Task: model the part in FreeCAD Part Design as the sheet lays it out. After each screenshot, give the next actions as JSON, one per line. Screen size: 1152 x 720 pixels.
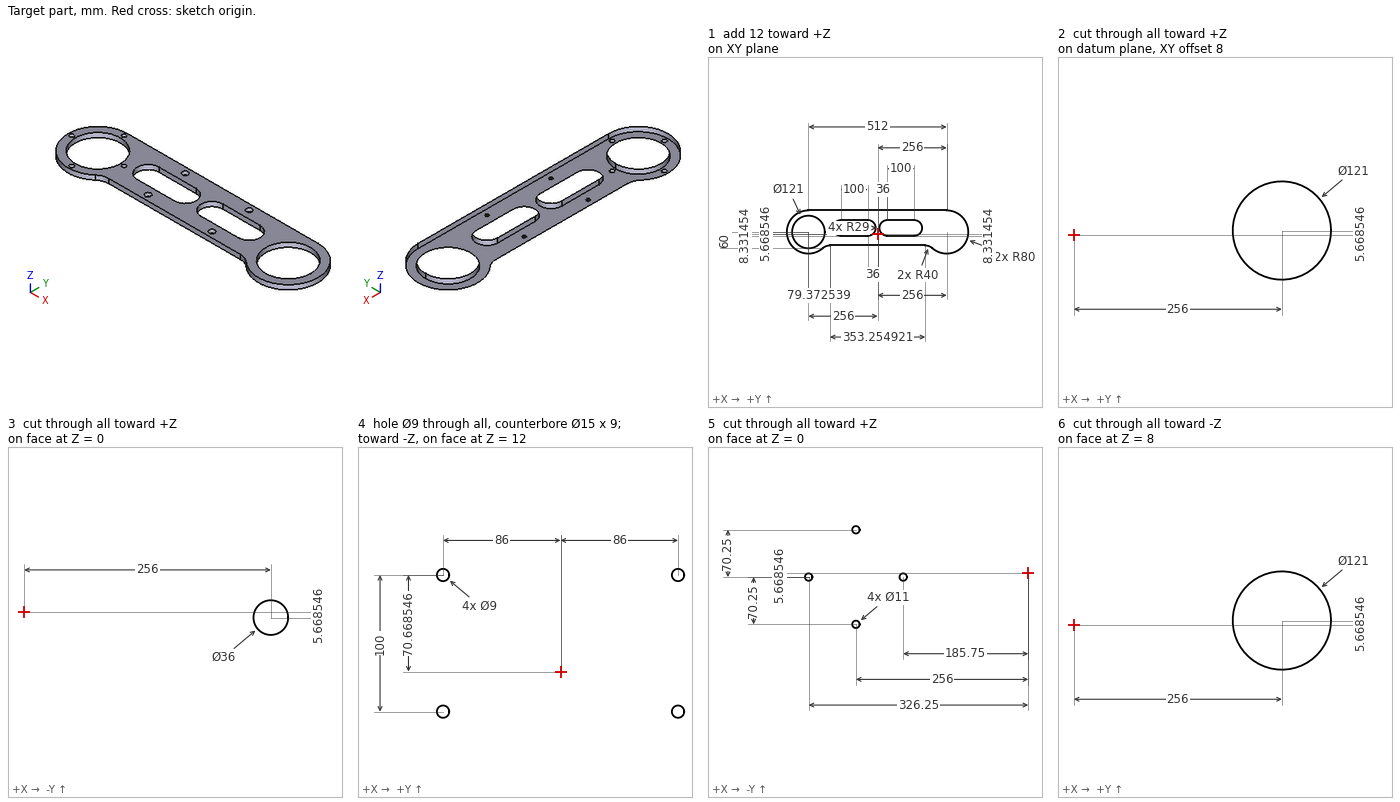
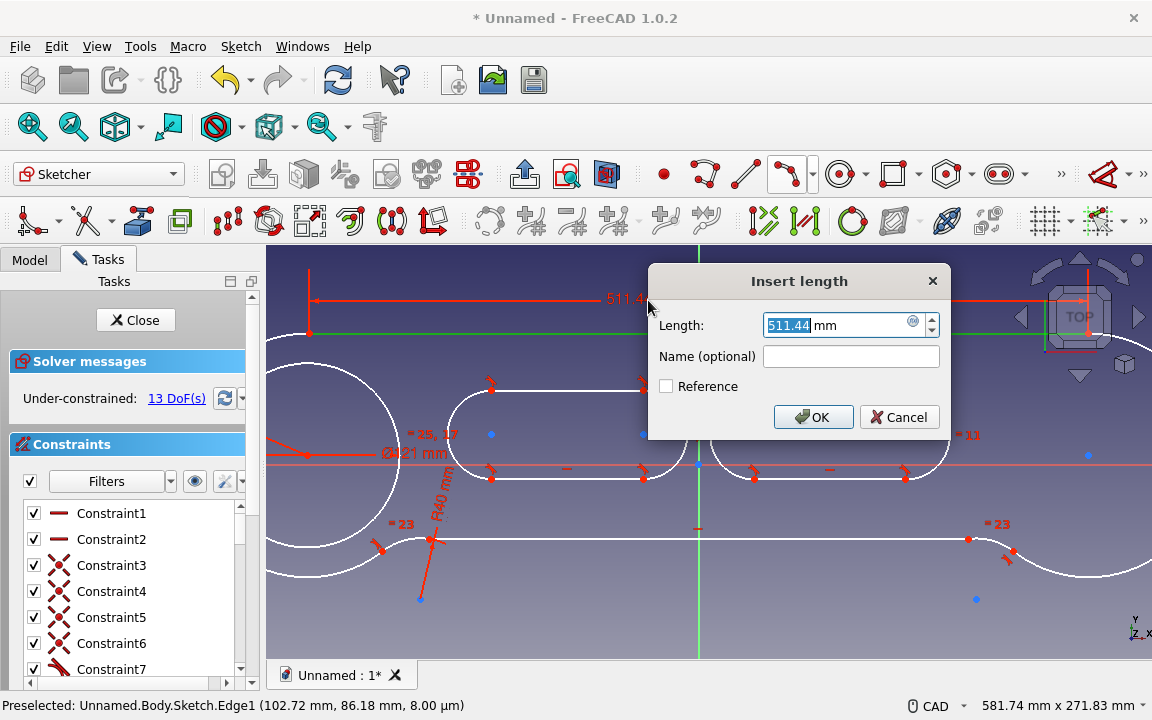
{"action": "type", "text": "512"}
{"action": "key", "text": "Return"}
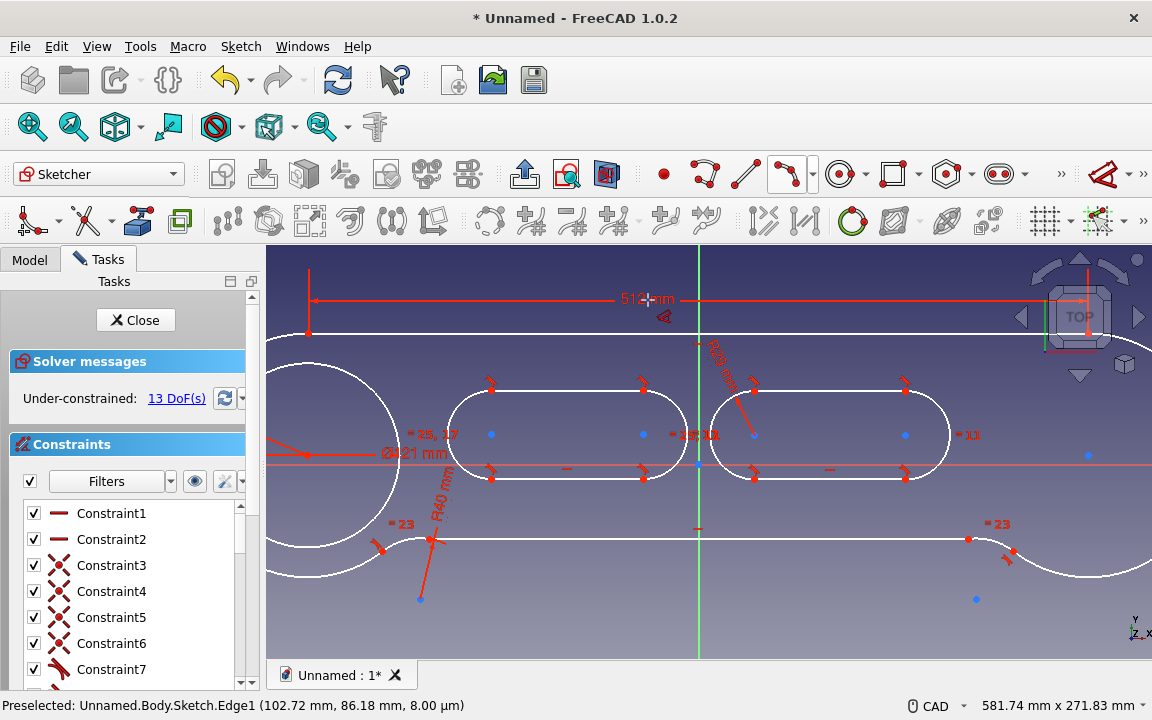
{"action": "left_click", "coordinate": [800, 391]}
{"action": "left_click", "coordinate": [830, 357]}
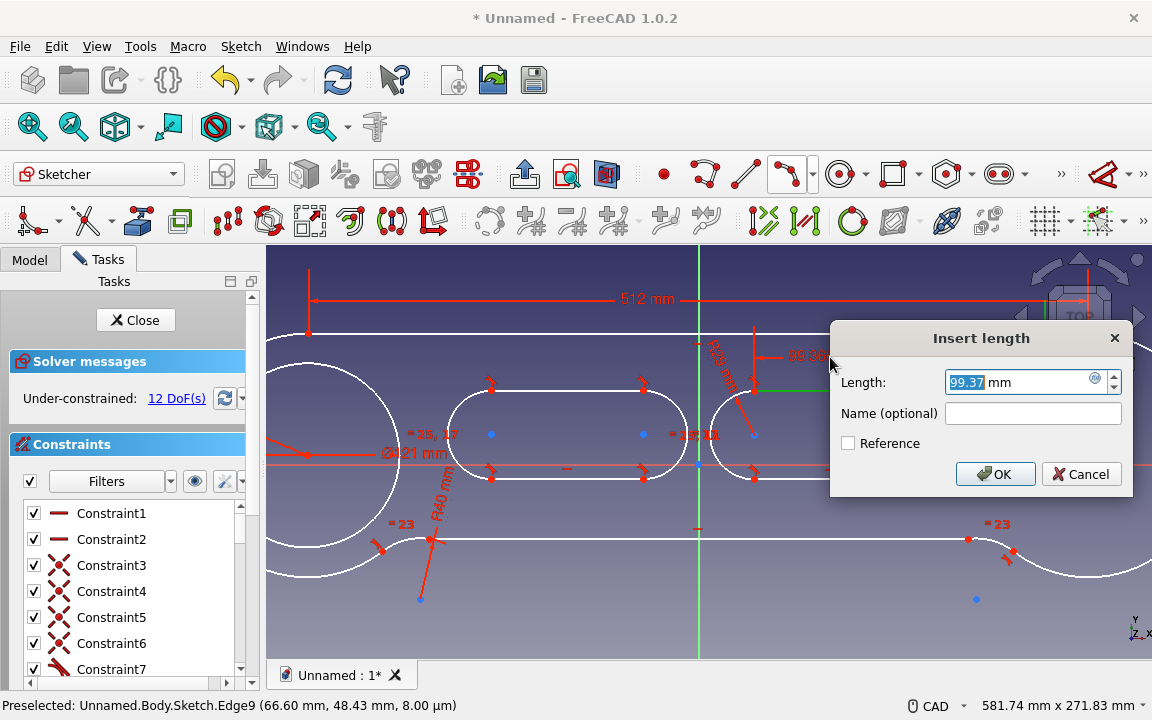
{"action": "type", "text": "100"}
{"action": "key", "text": "Return"}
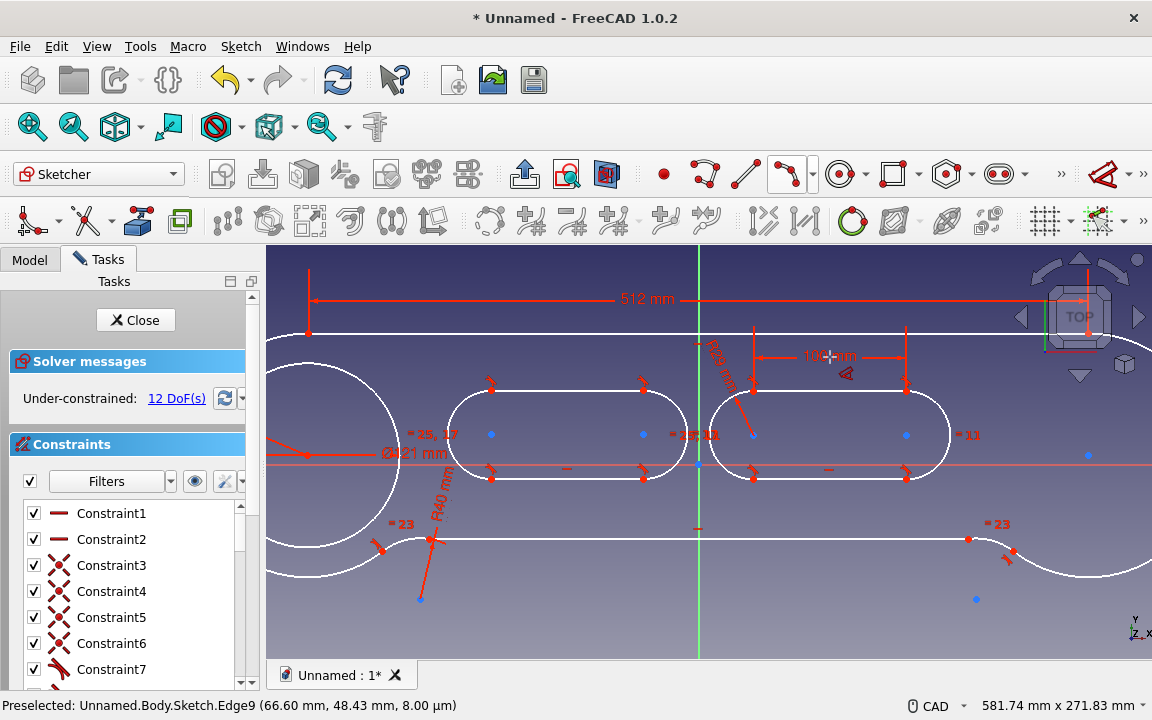
{"action": "left_click", "coordinate": [537, 391]}
{"action": "left_click", "coordinate": [567, 357]}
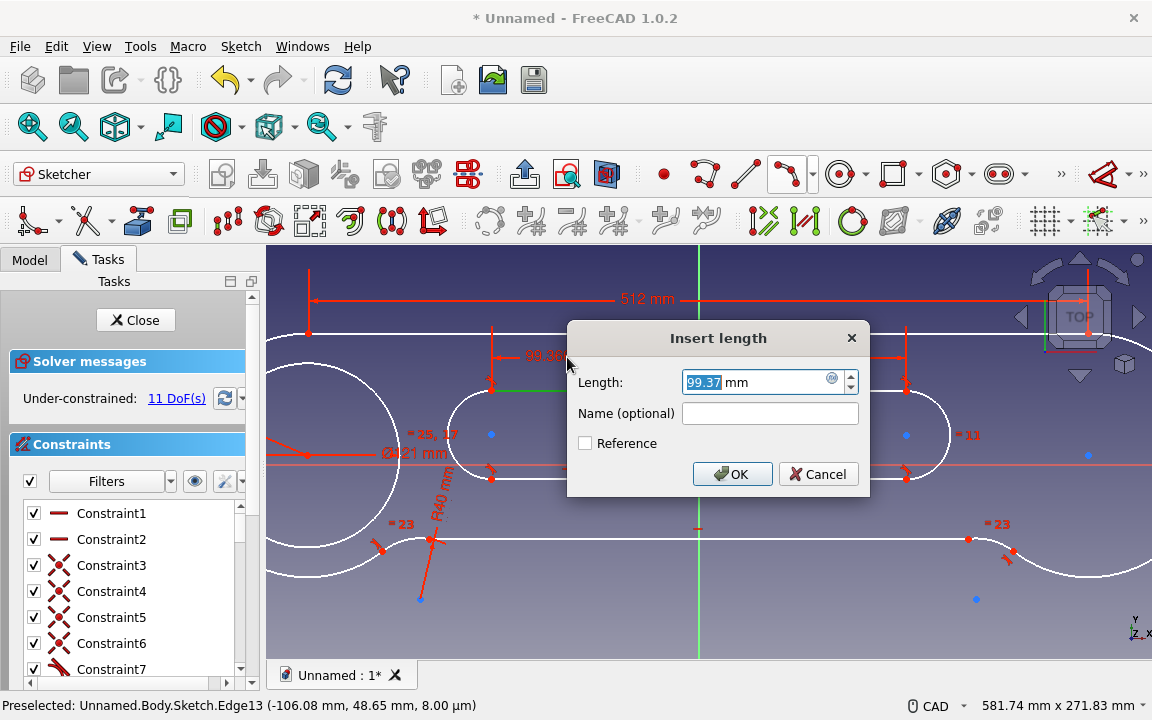
{"action": "type", "text": "100"}
{"action": "key", "text": "Return"}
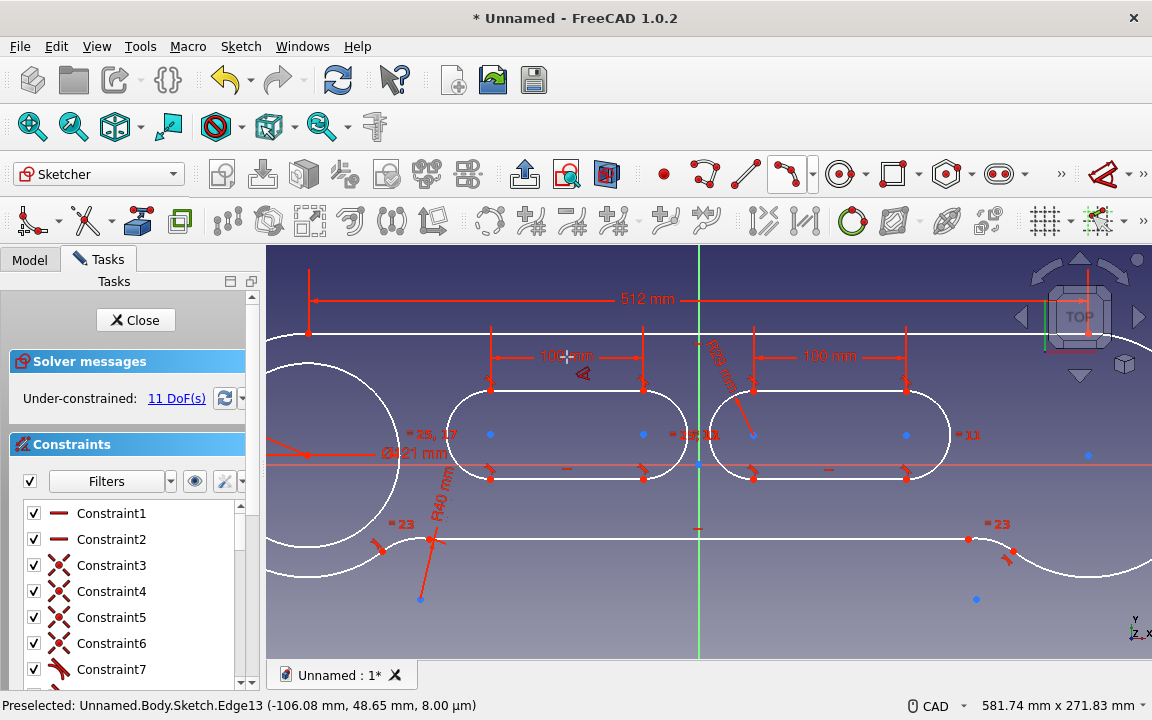
{"action": "left_click", "coordinate": [754, 391]}
{"action": "left_click", "coordinate": [726, 499]}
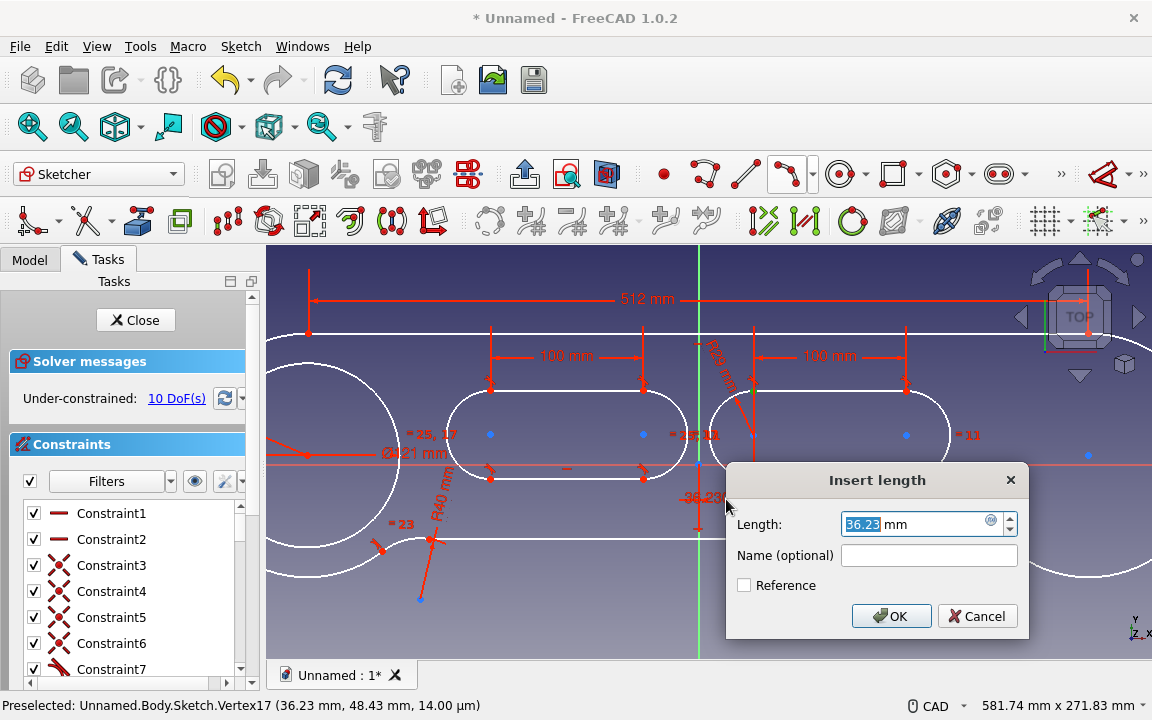
{"action": "type", "text": "36"}
{"action": "key", "text": "Return"}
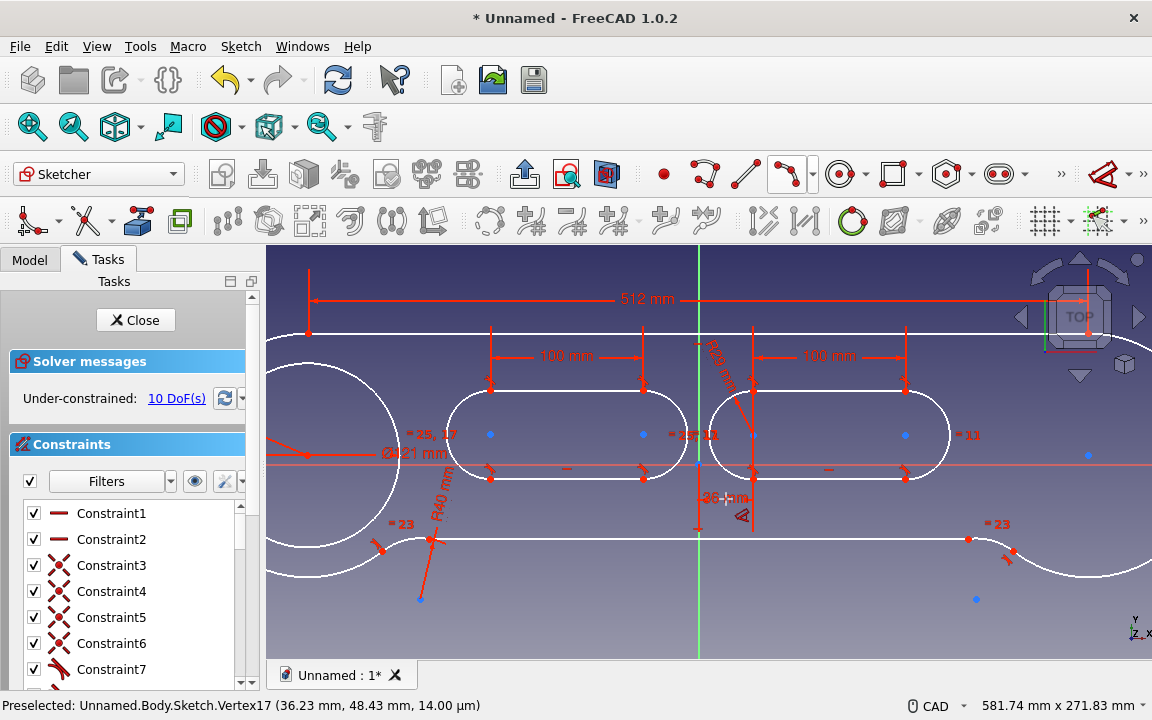
{"action": "left_click", "coordinate": [643, 479]}
{"action": "left_click", "coordinate": [652, 513]}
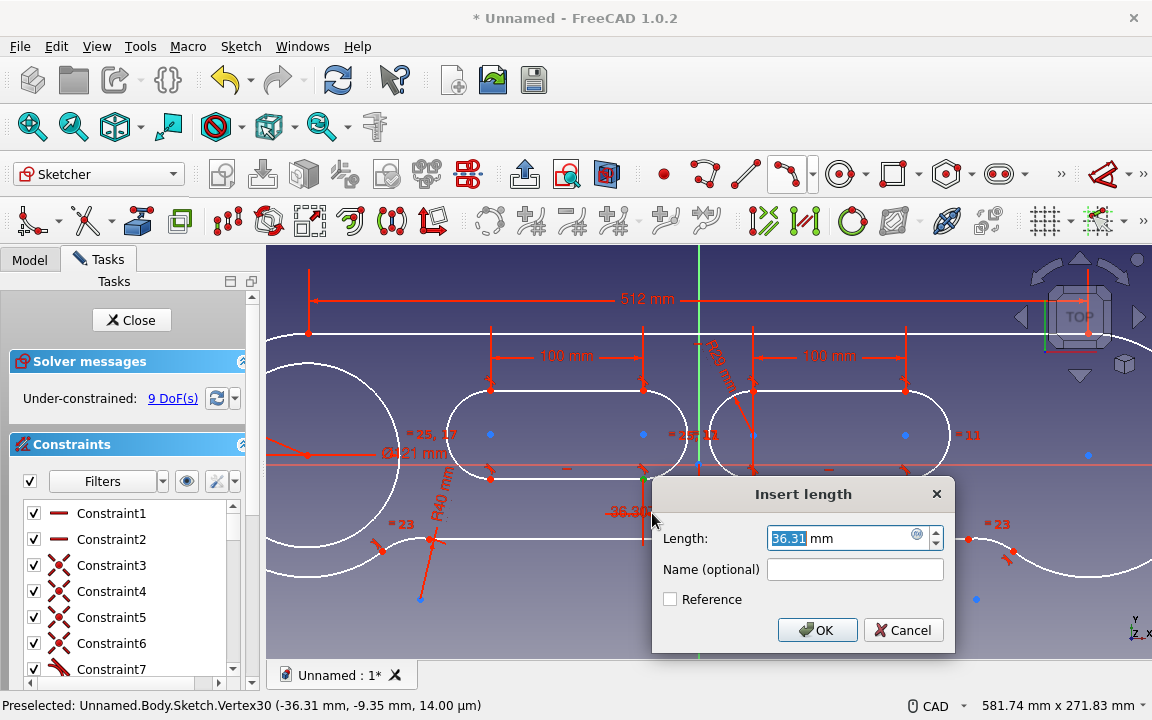
{"action": "type", "text": "36"}
{"action": "key", "text": "Return"}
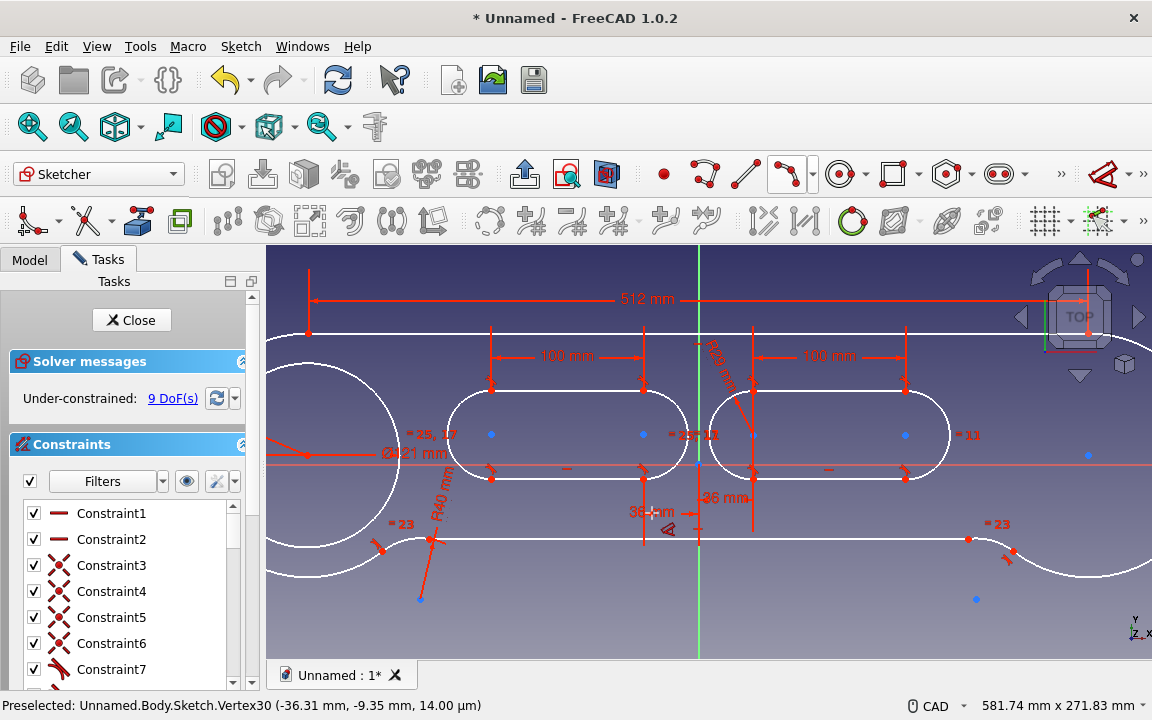
{"action": "left_click", "coordinate": [307, 455]}
{"action": "left_click", "coordinate": [366, 499]}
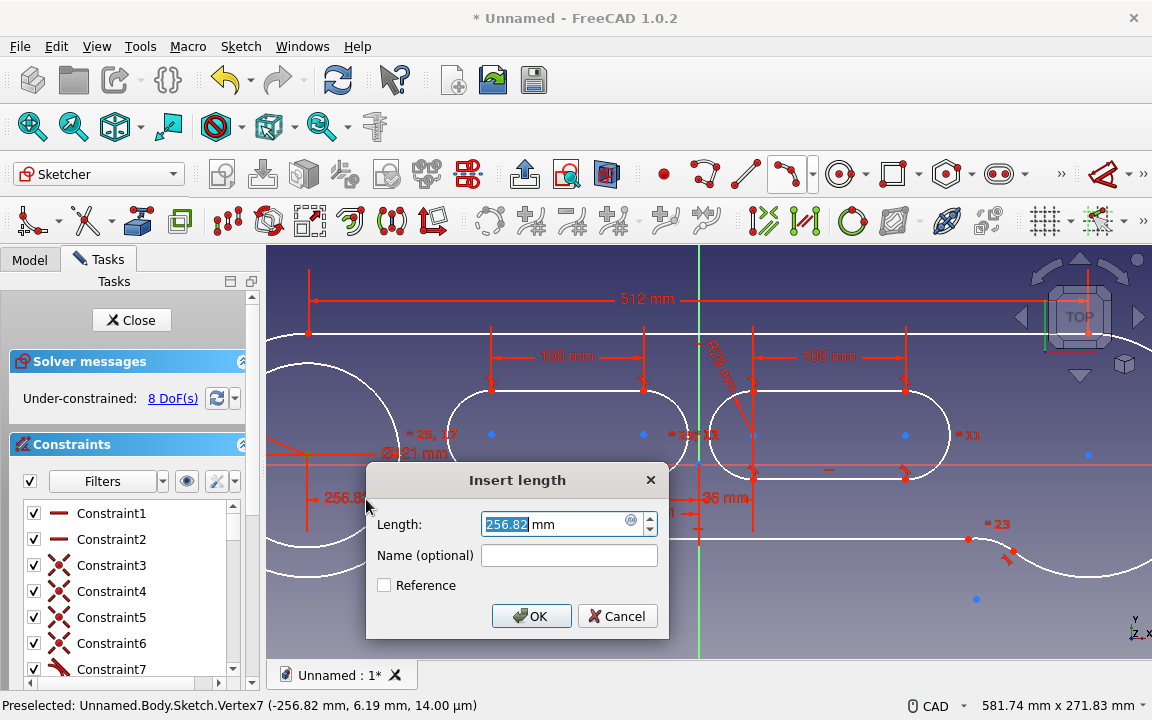
{"action": "type", "text": "256"}
{"action": "key", "text": "Return"}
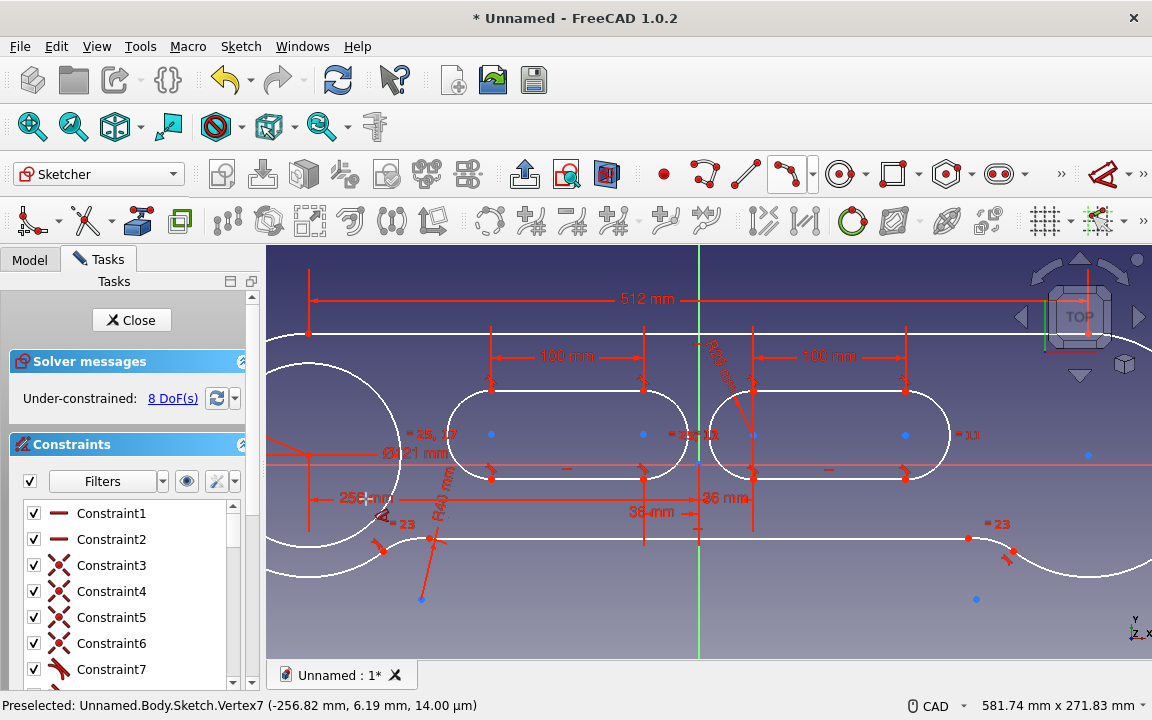
{"action": "left_click", "coordinate": [384, 551]}